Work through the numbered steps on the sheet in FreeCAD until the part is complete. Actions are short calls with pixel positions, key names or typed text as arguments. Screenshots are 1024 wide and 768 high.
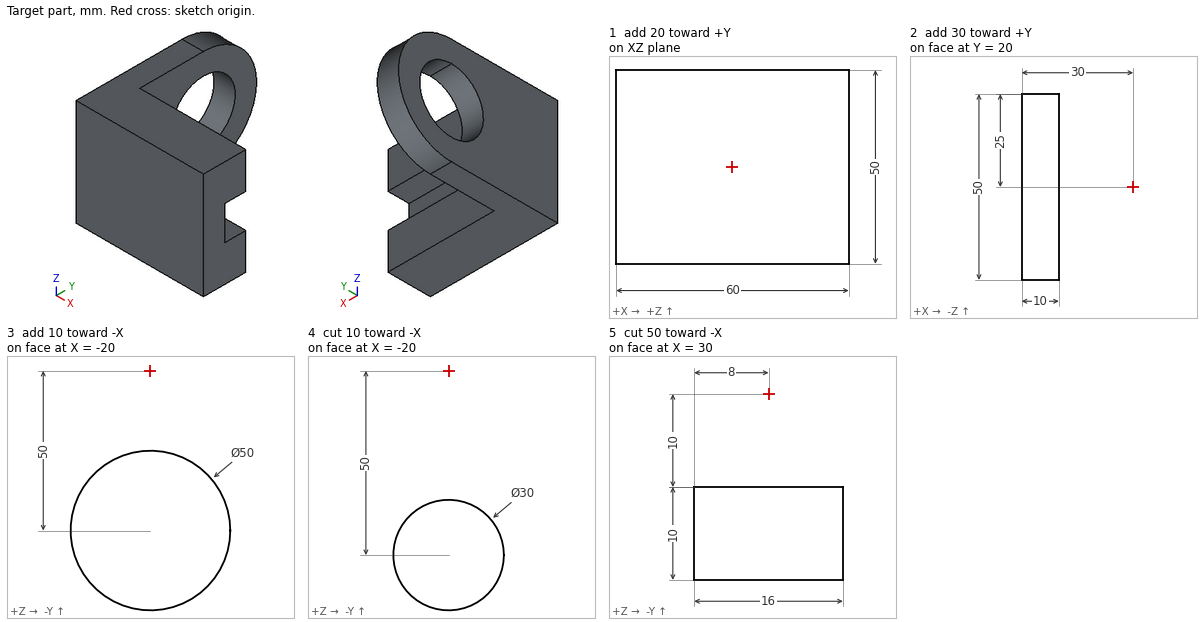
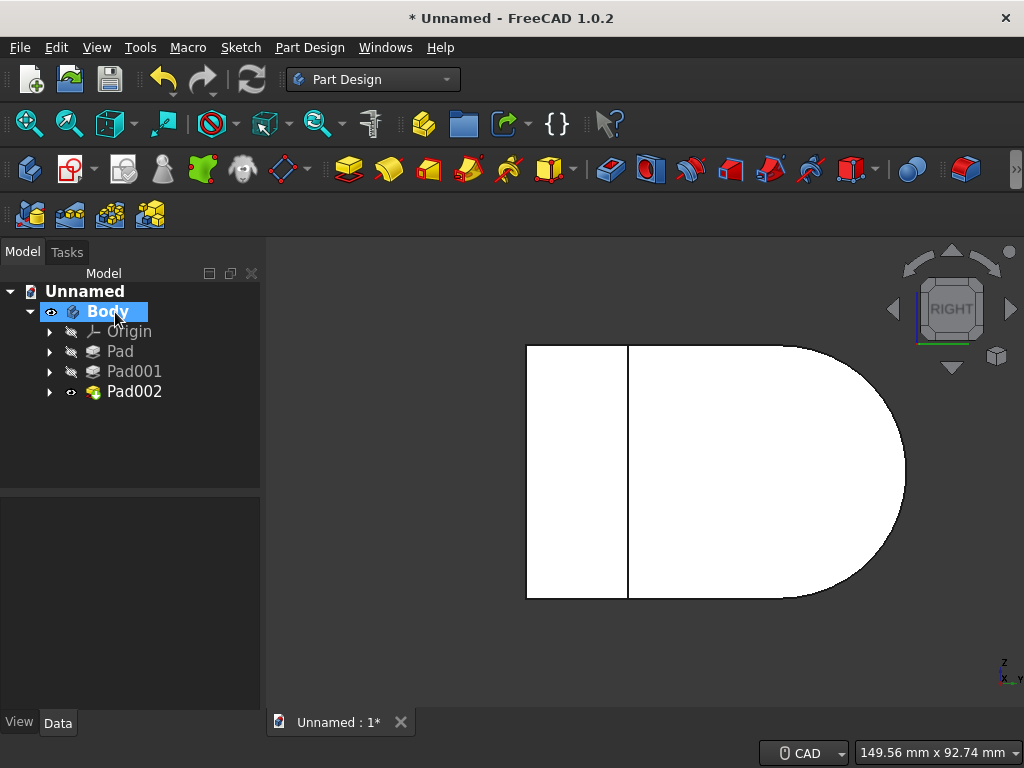
click(767, 471)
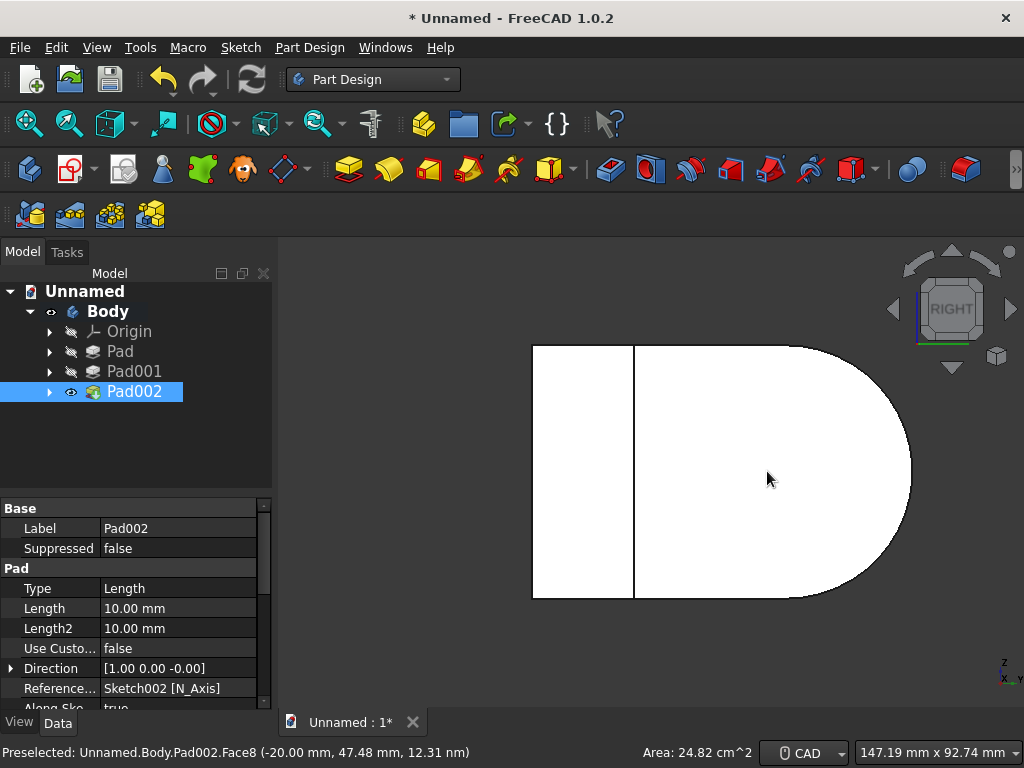
click(70, 170)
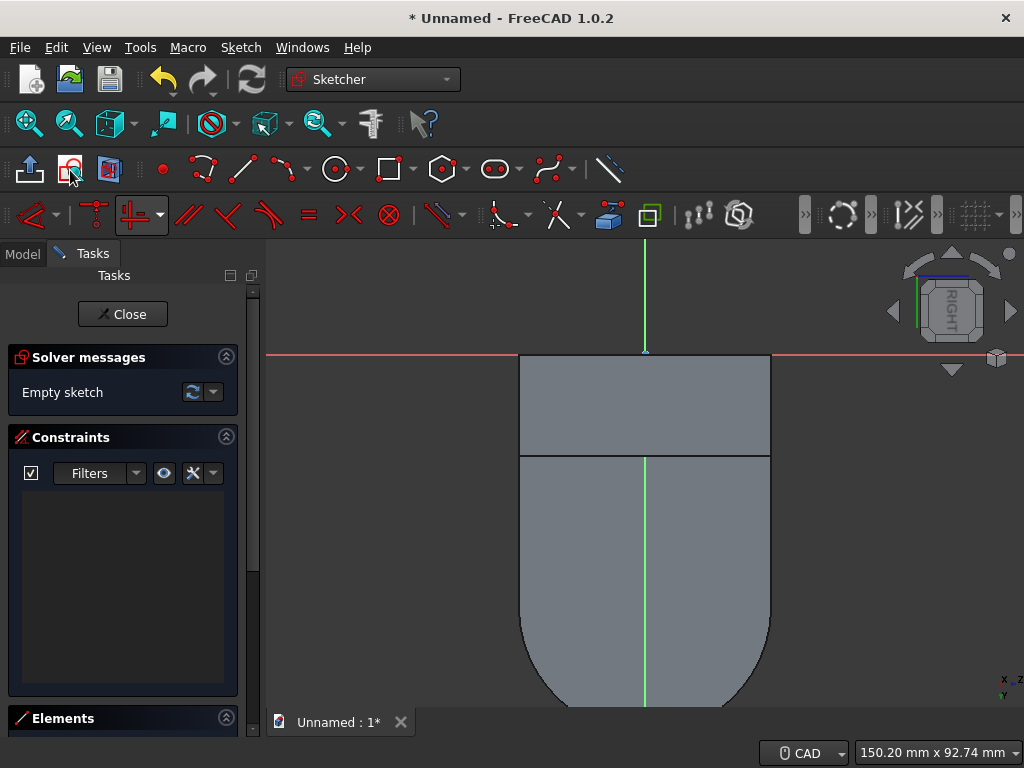
key(q)
key(s)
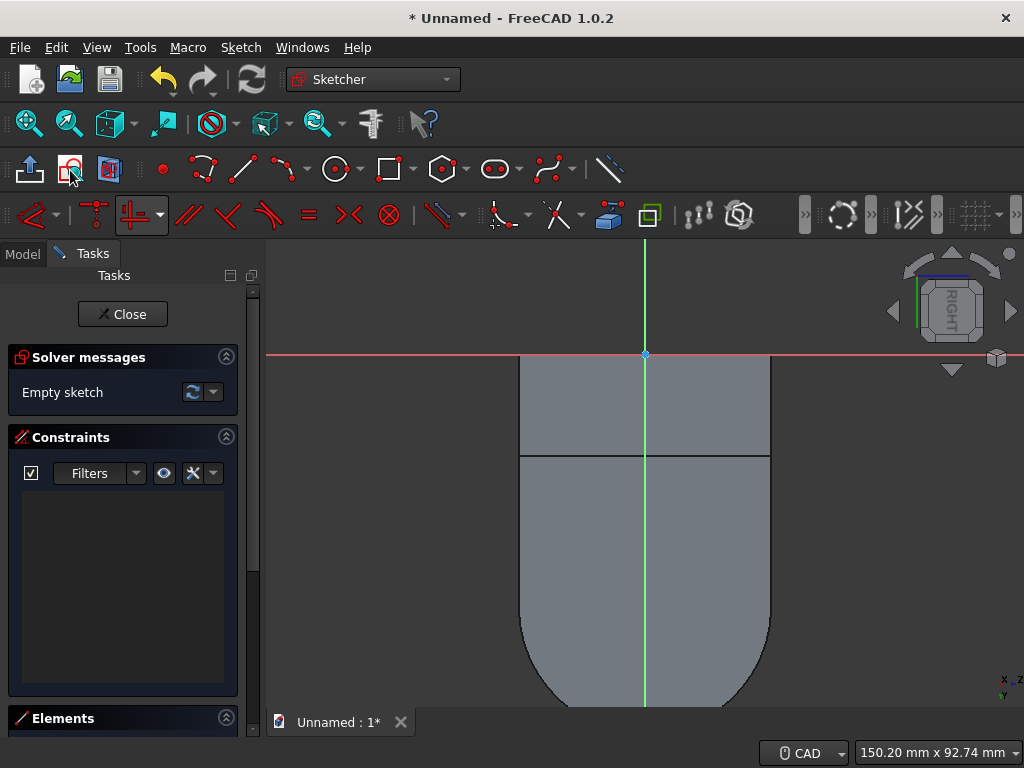
scroll(294, 267, down, 1)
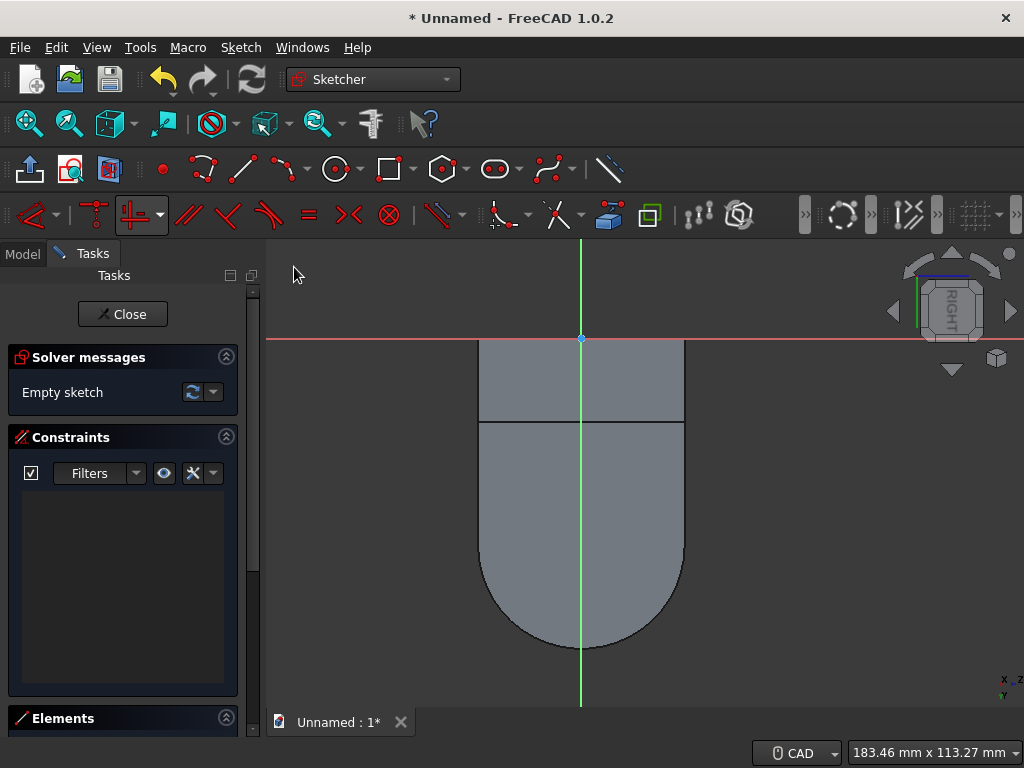
click(336, 170)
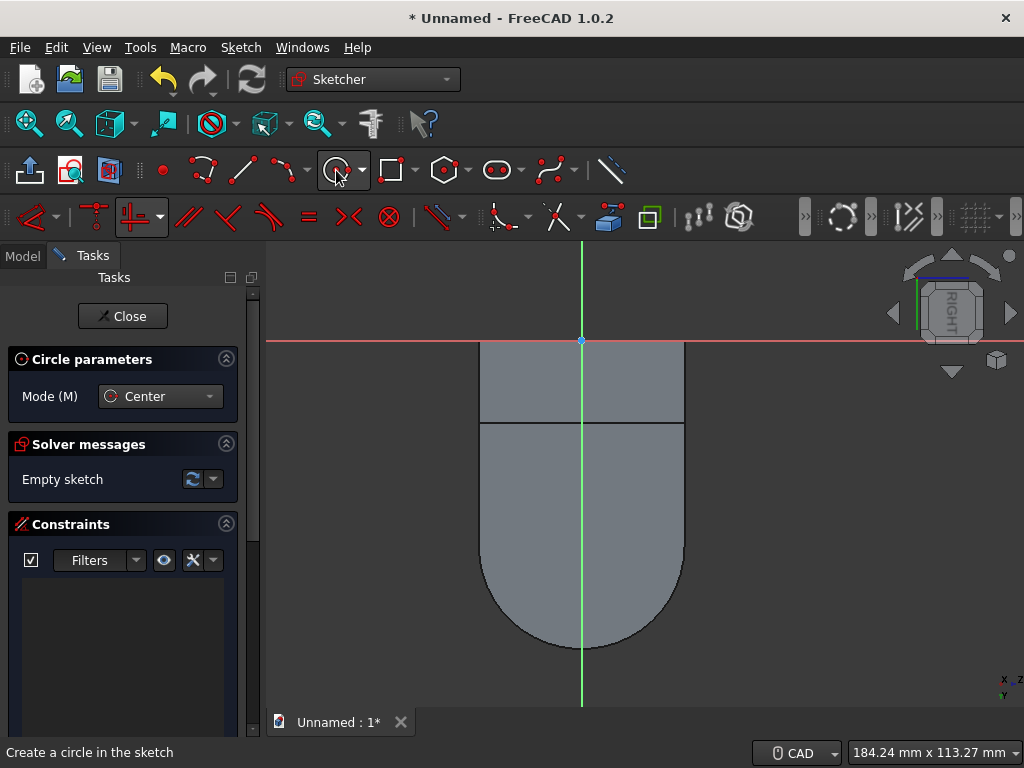
click(582, 546)
click(625, 503)
key(Escape)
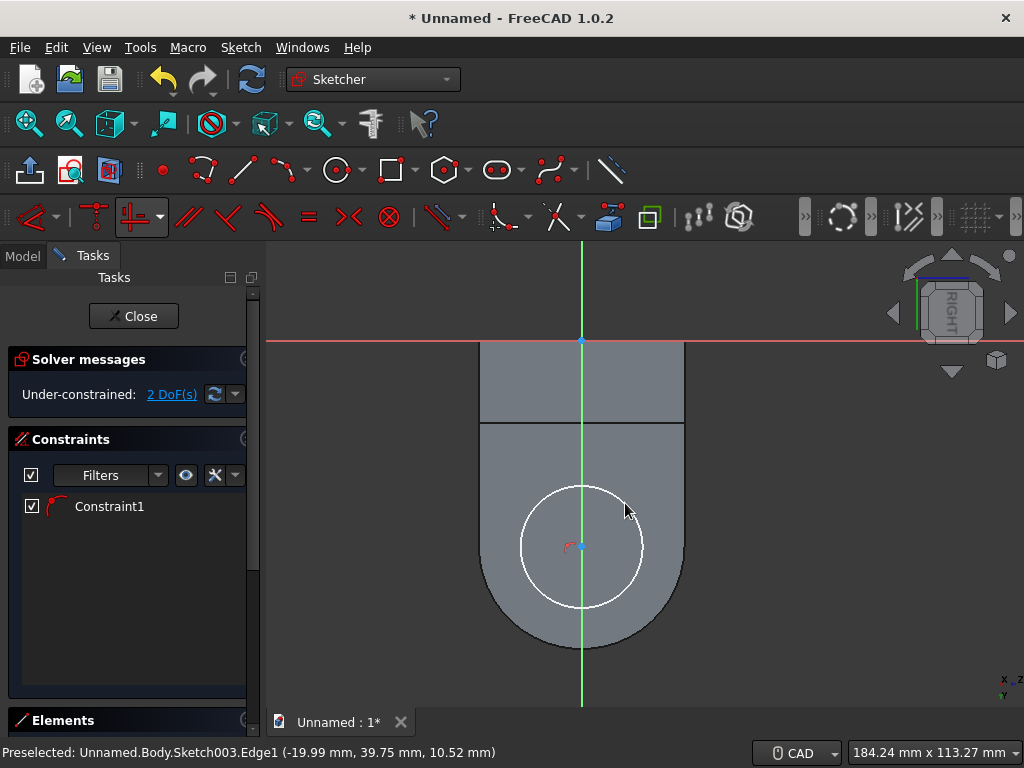
click(32, 218)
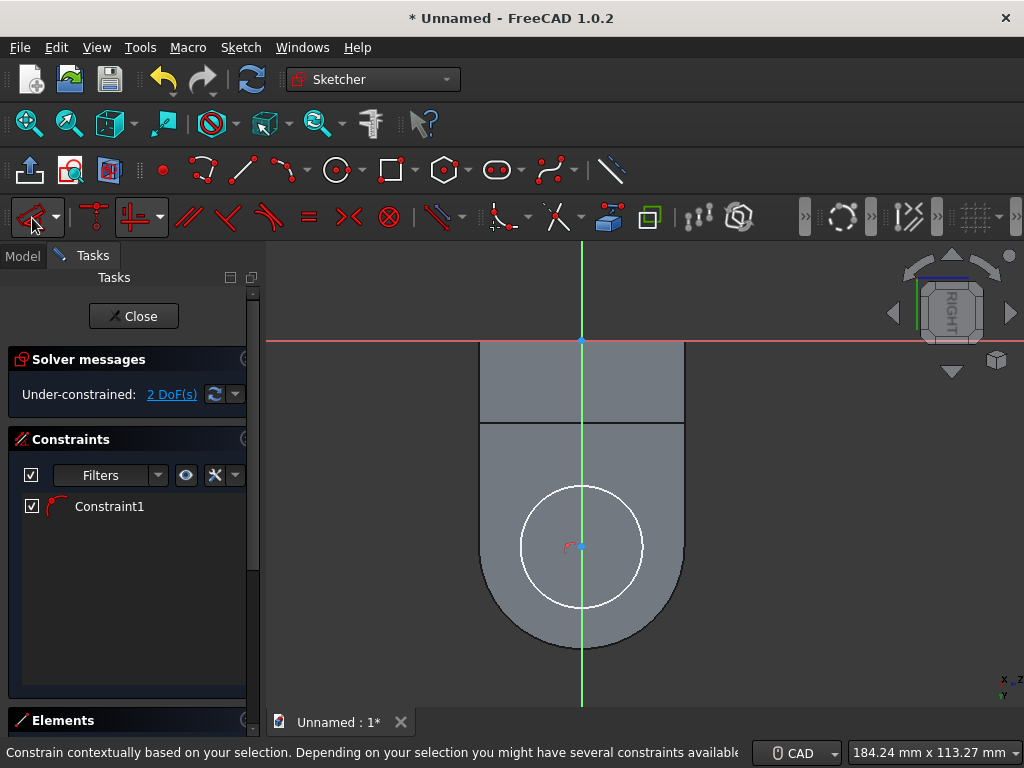
click(625, 504)
click(648, 481)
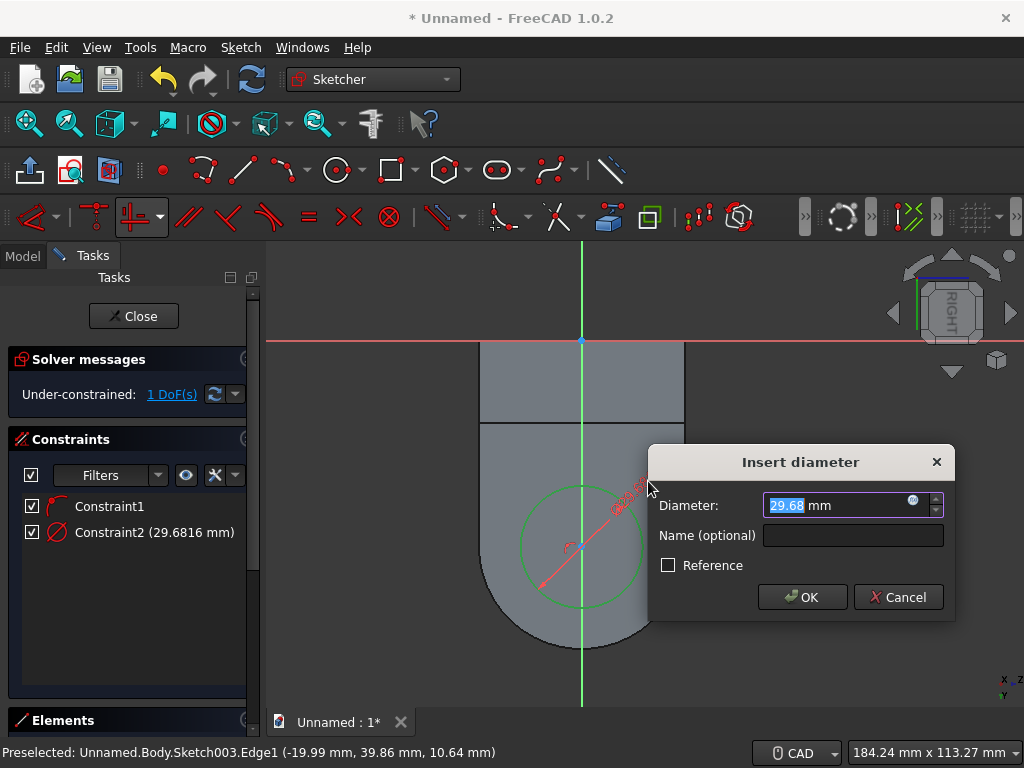
text(30)
key(Return)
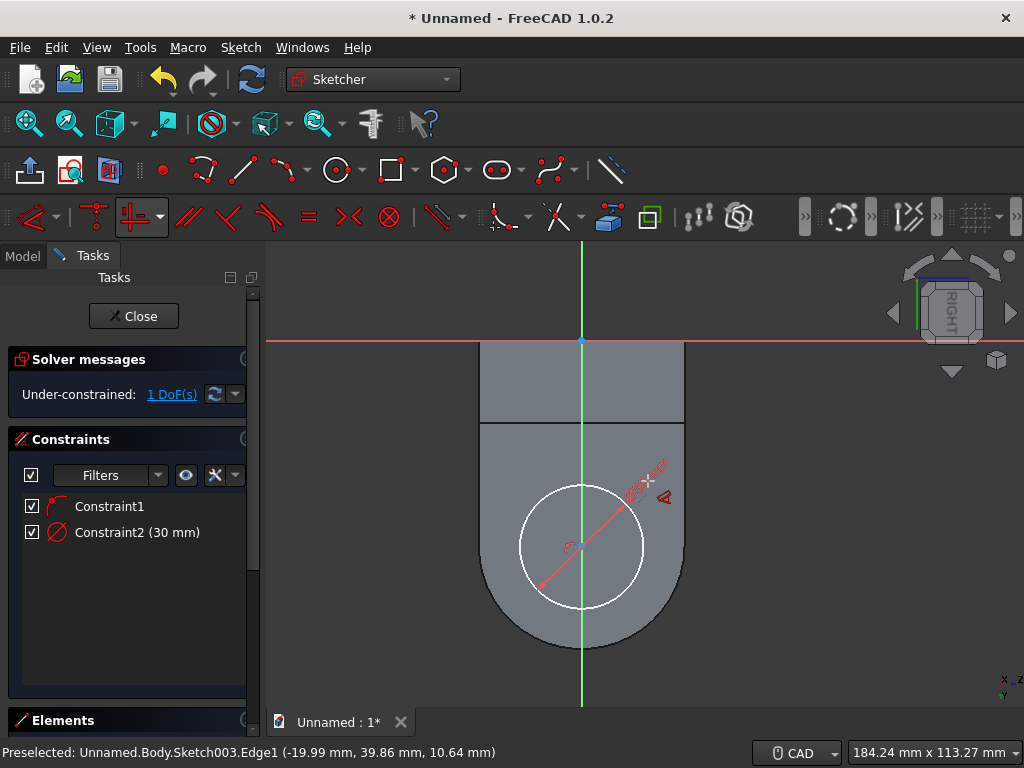
click(582, 547)
click(616, 444)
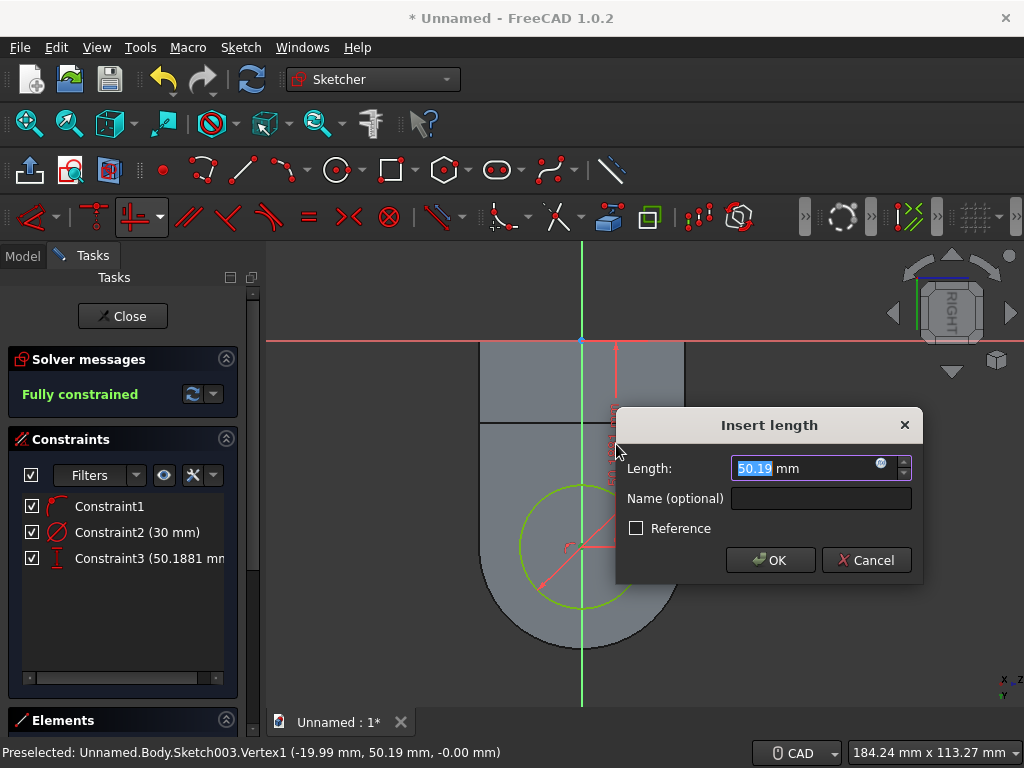
text(50)
key(Return)
key(Escape)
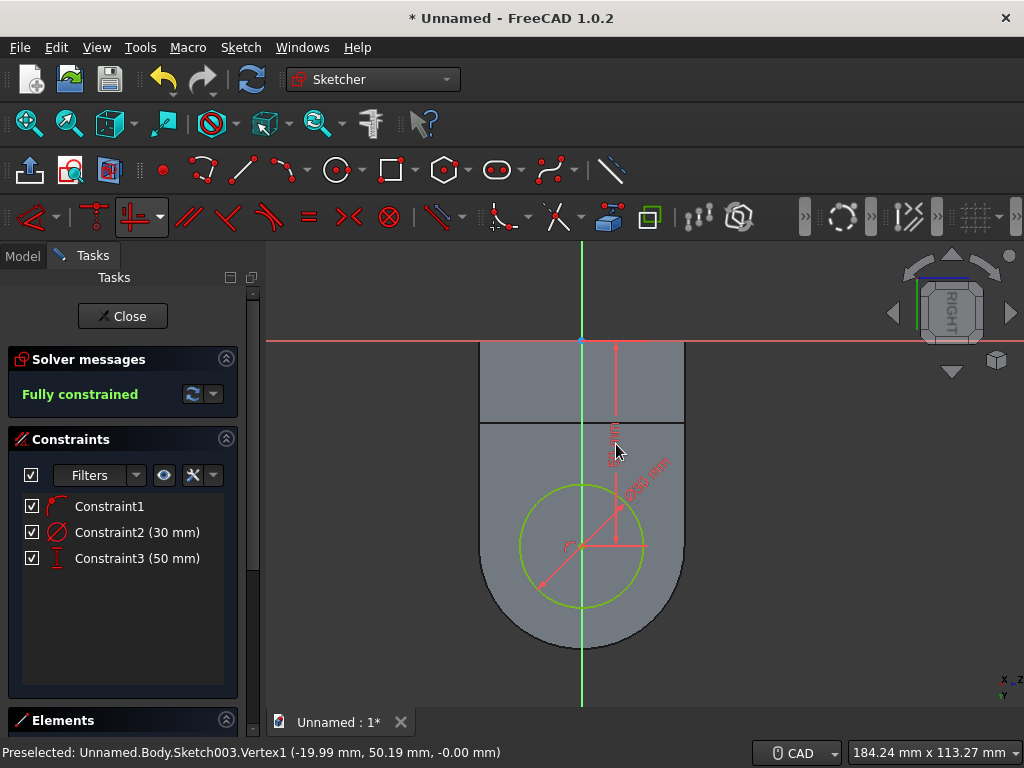
click(123, 316)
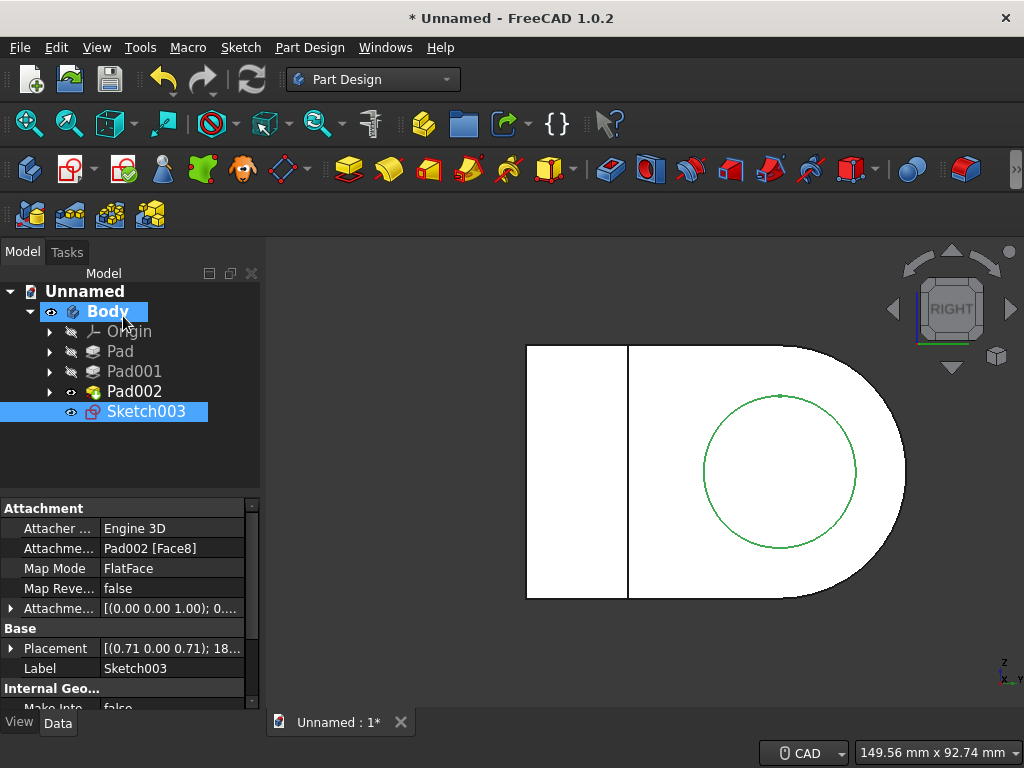
click(612, 170)